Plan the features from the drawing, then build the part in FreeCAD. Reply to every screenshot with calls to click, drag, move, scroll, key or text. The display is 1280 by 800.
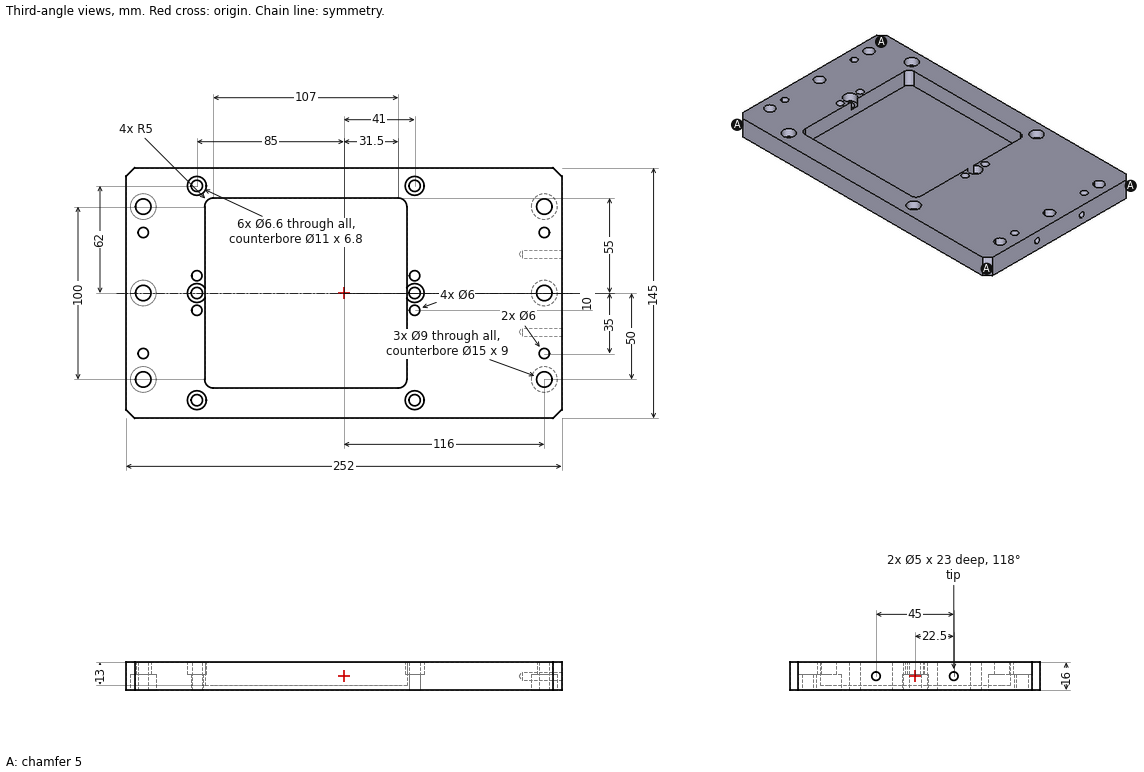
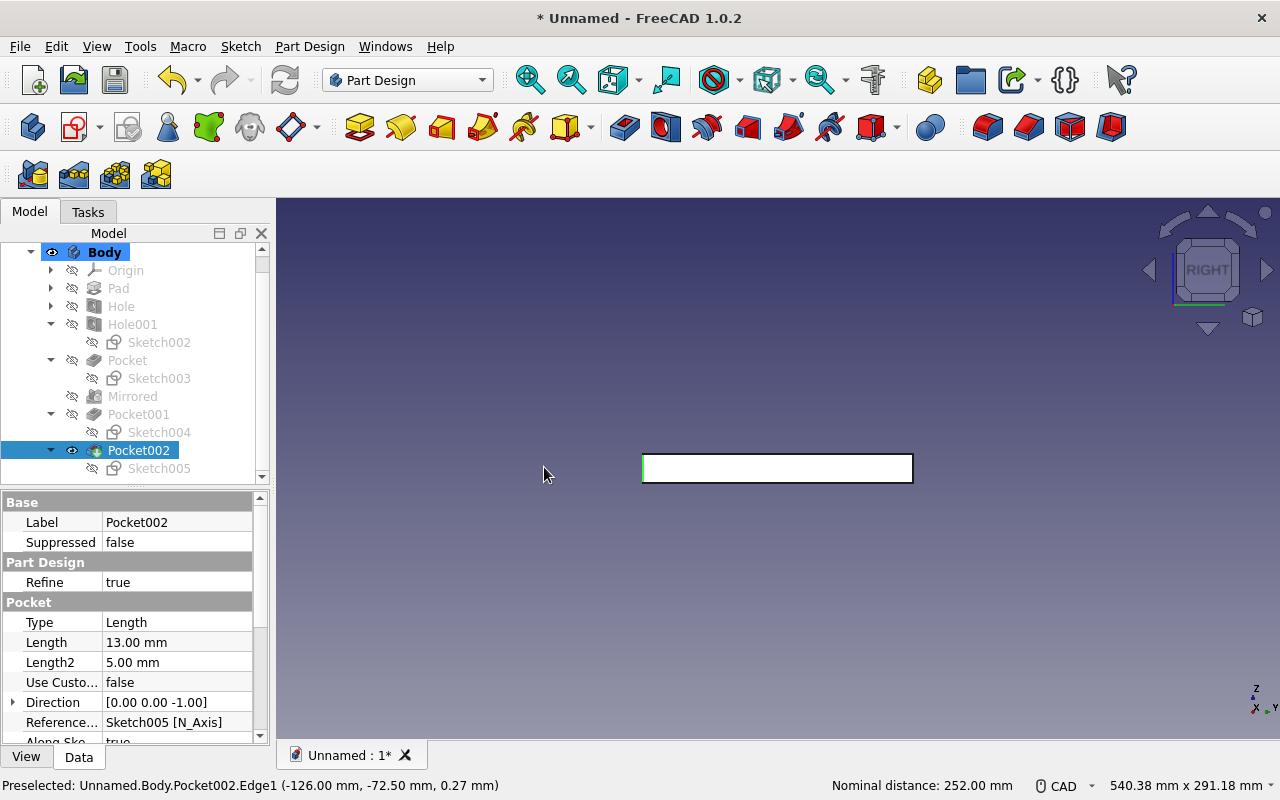
key(v)
key(f)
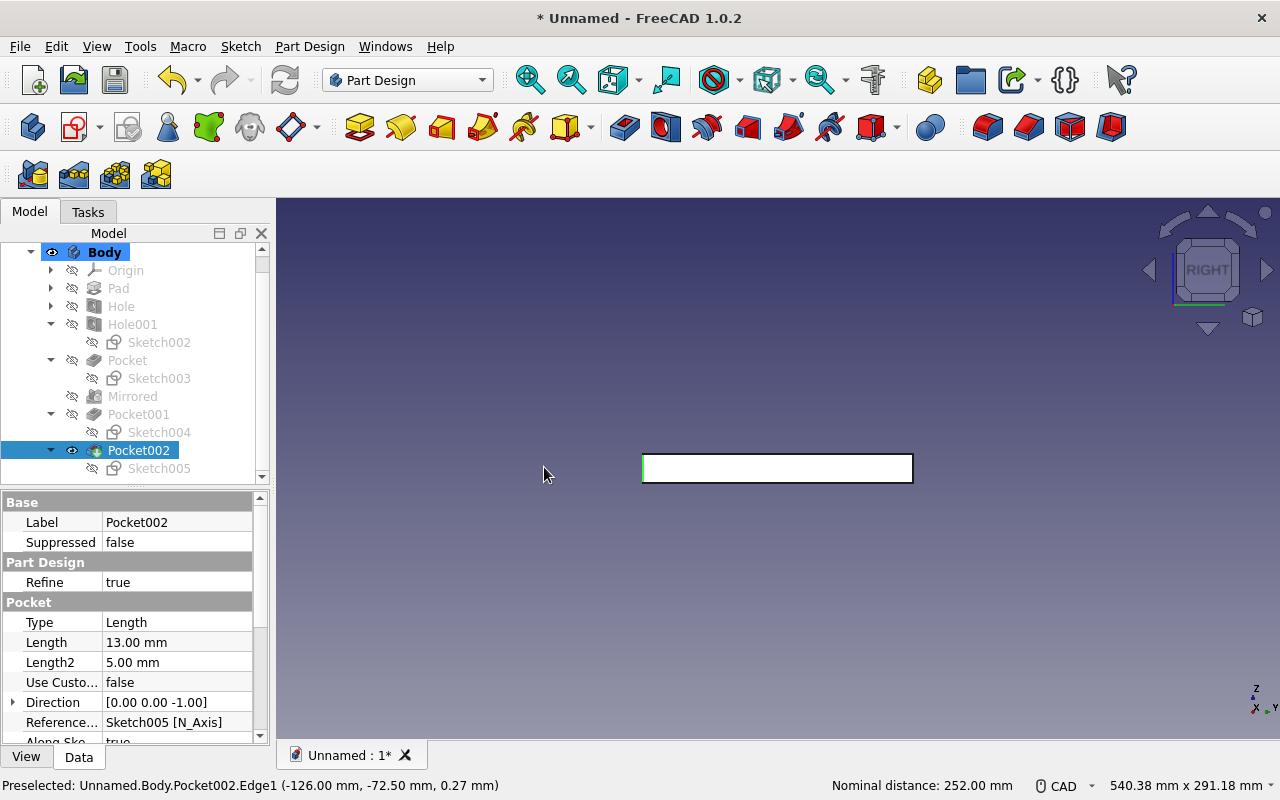
click(913, 467, ctrl)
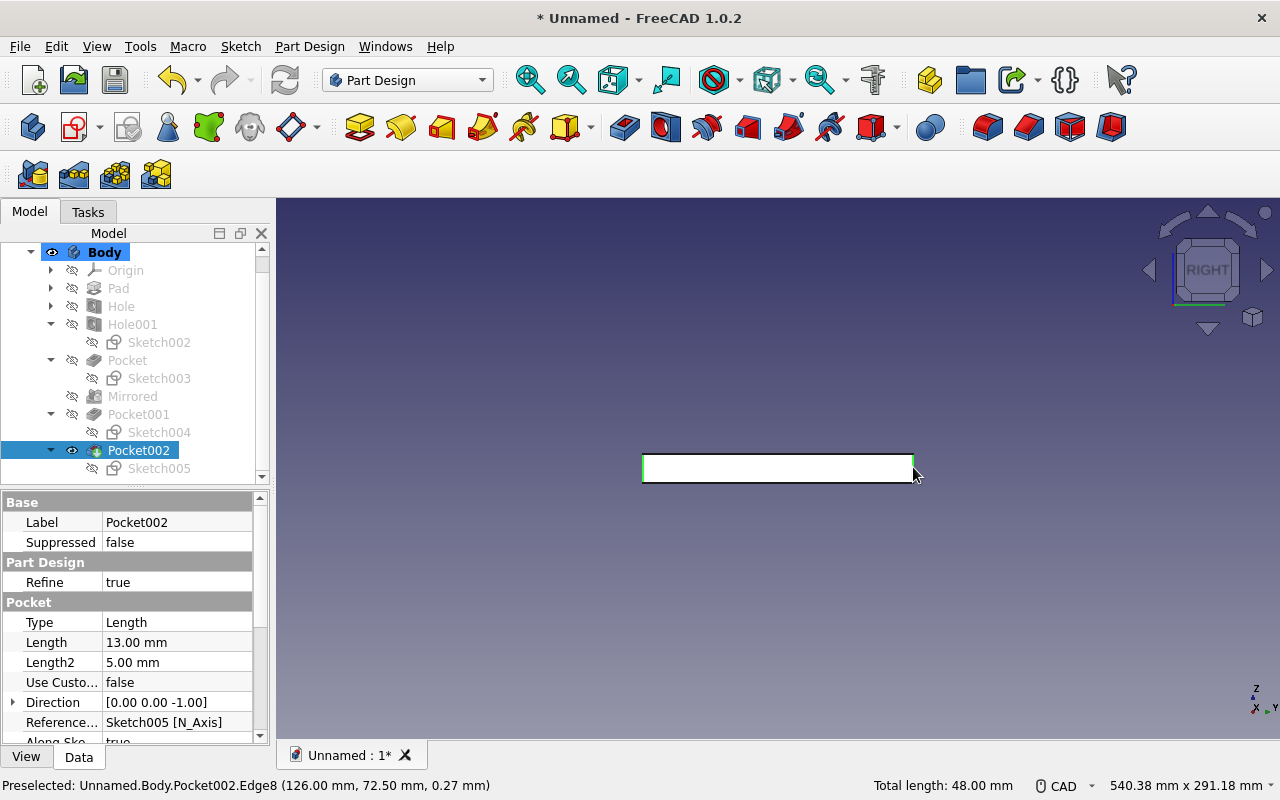
key(5)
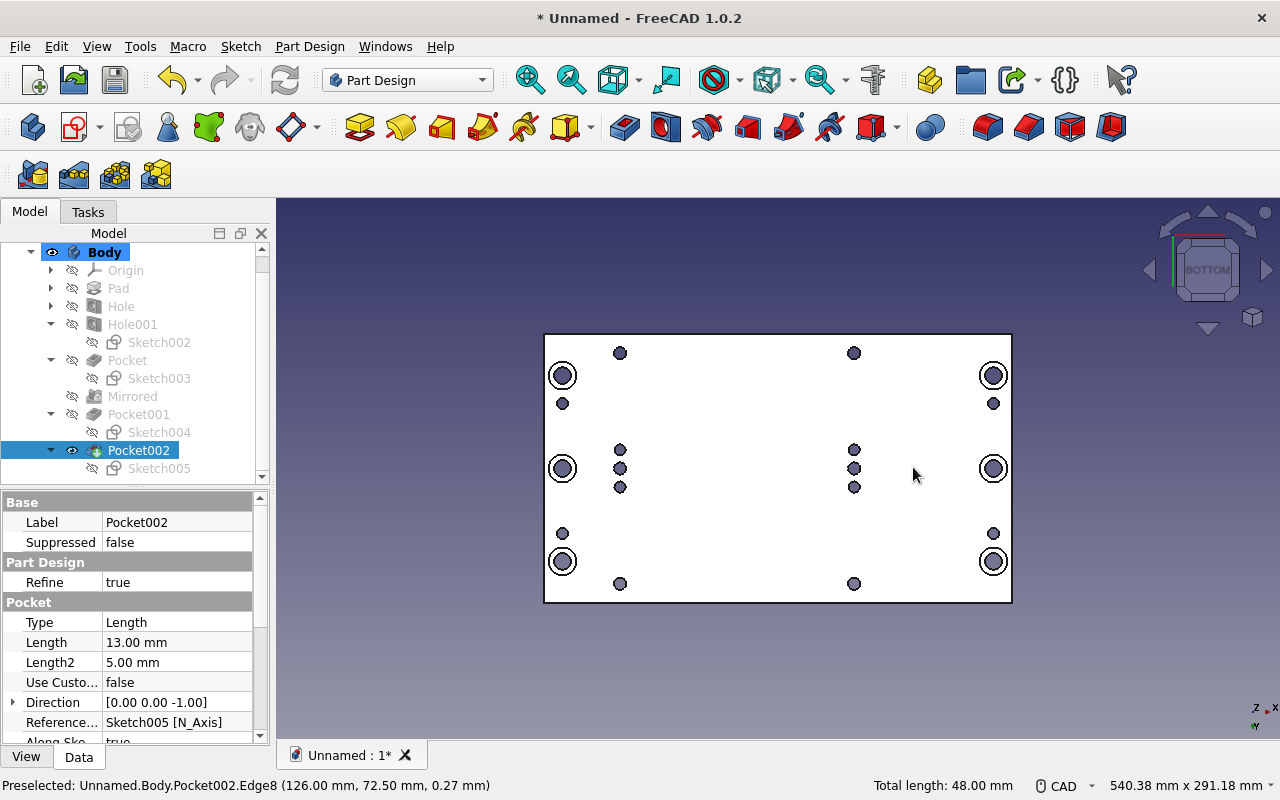
key(4)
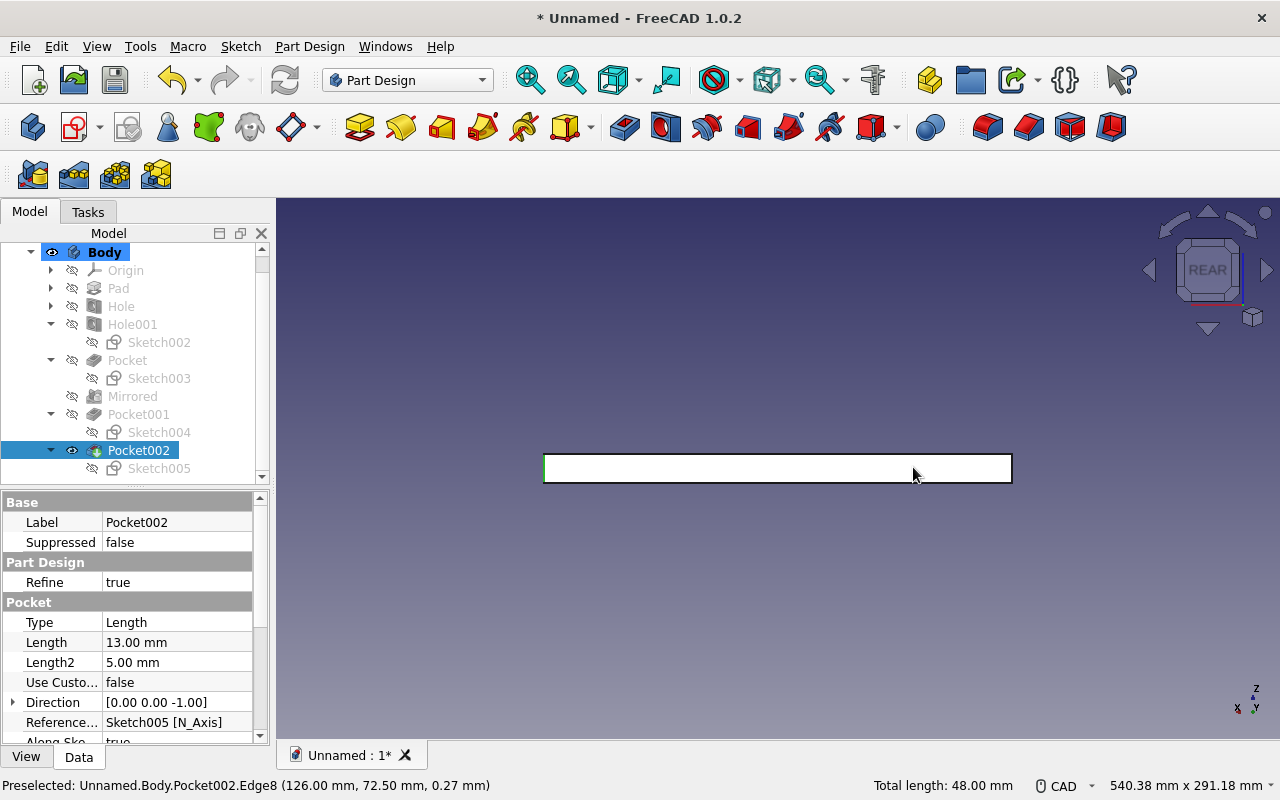
click(1012, 467, ctrl)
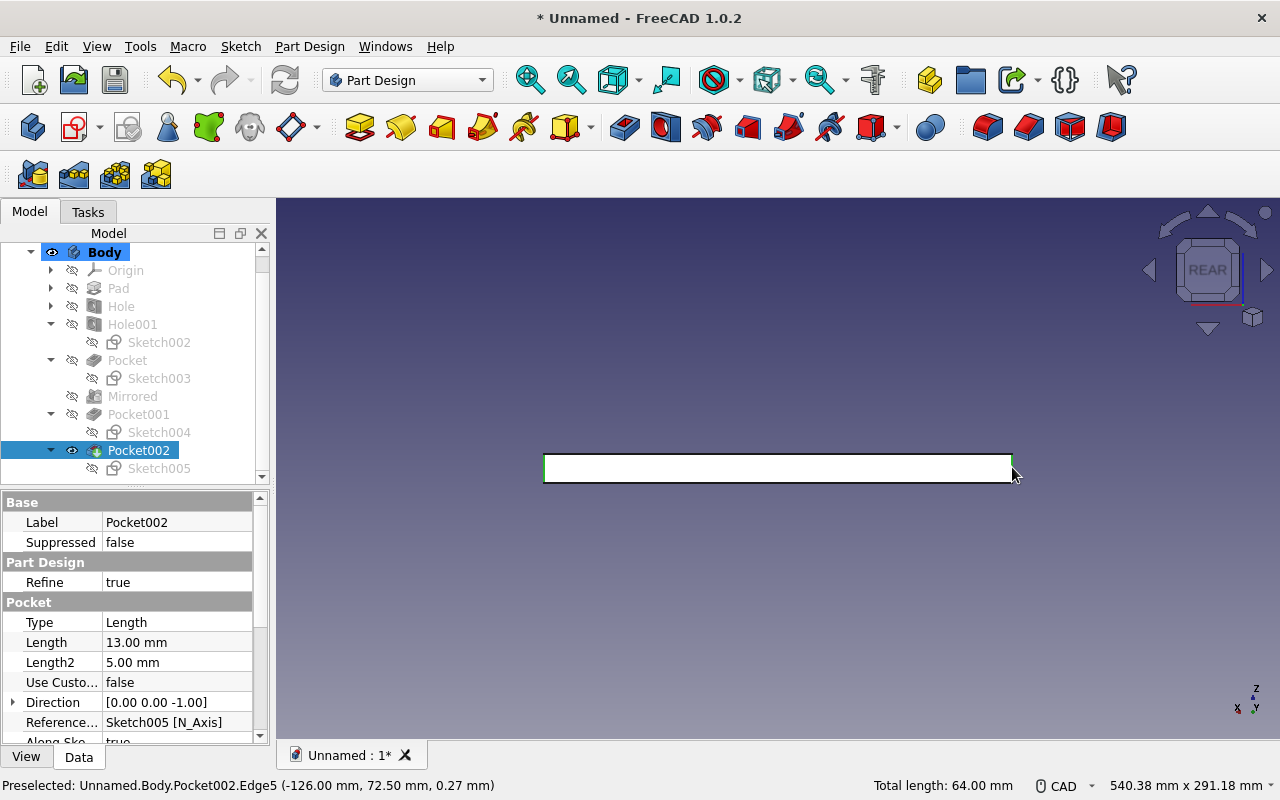
click(1029, 128)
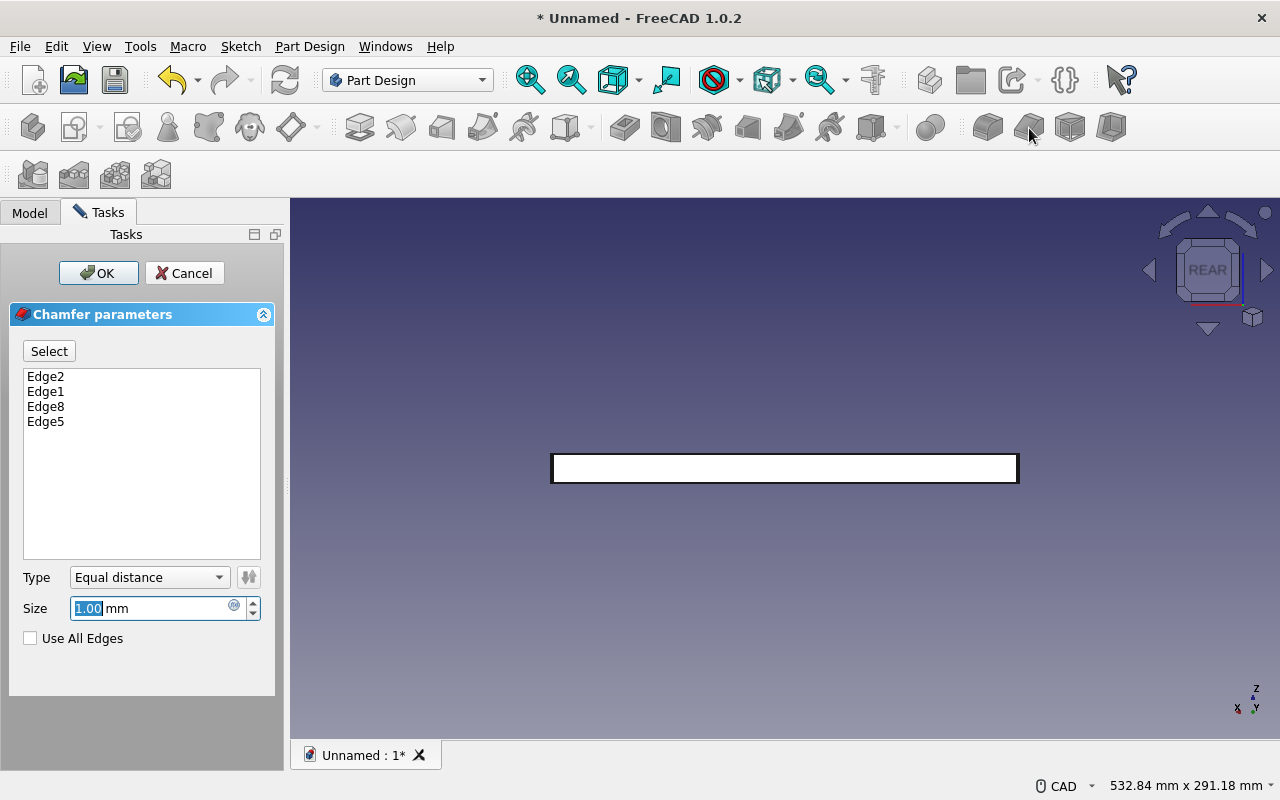
text(5)
key(Tab)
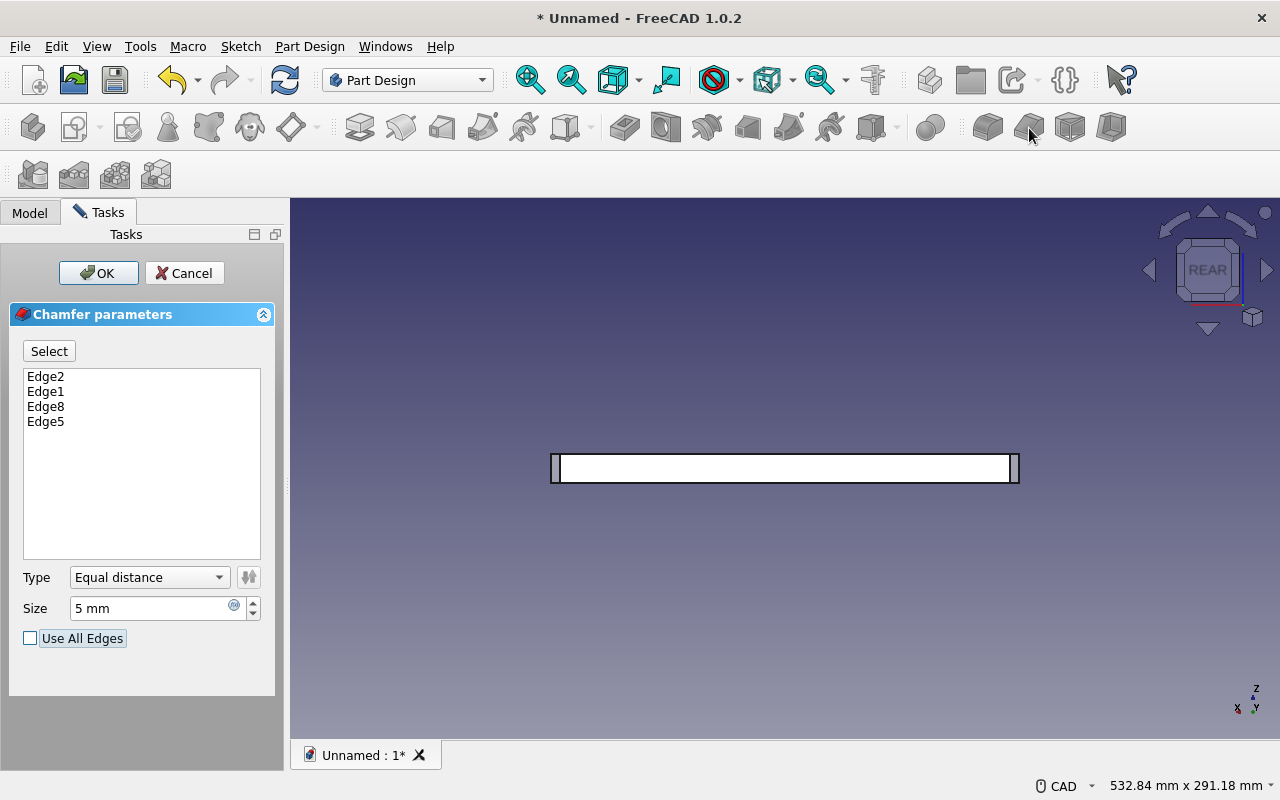
click(99, 273)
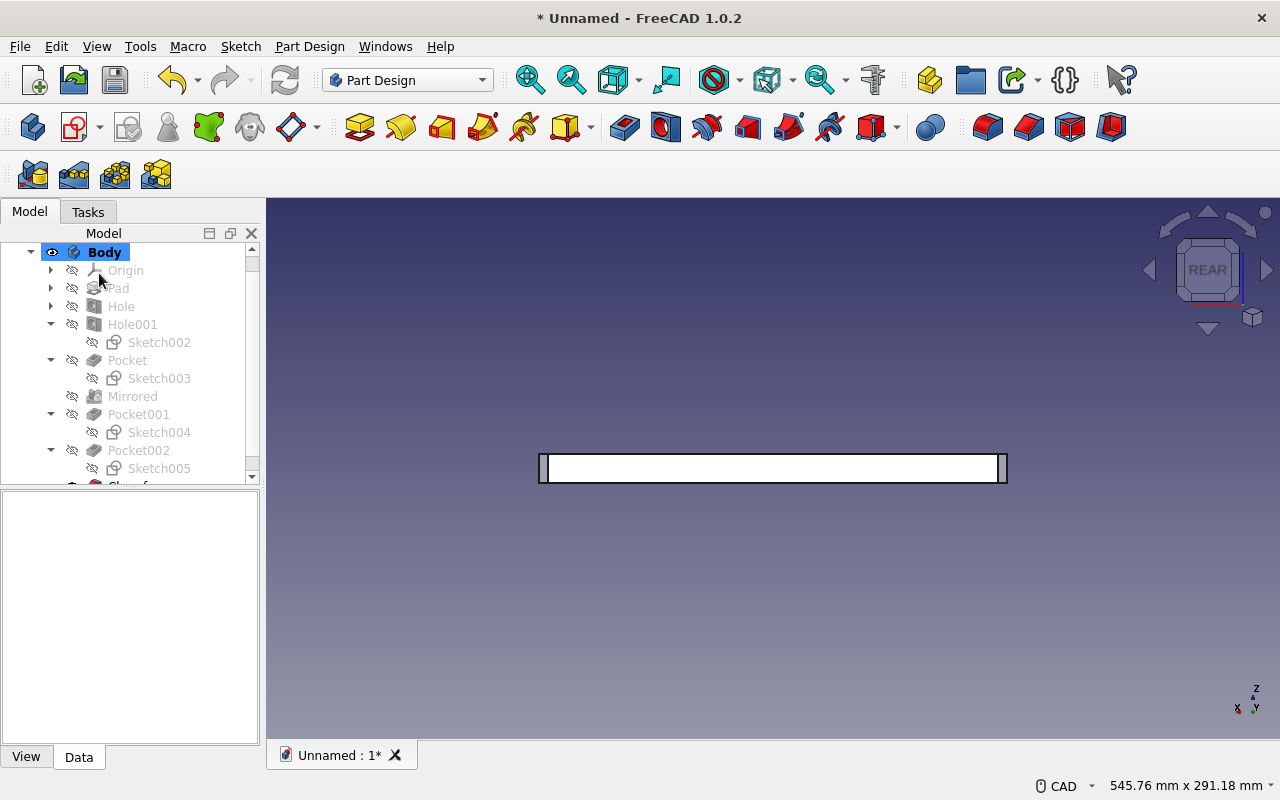
key(0)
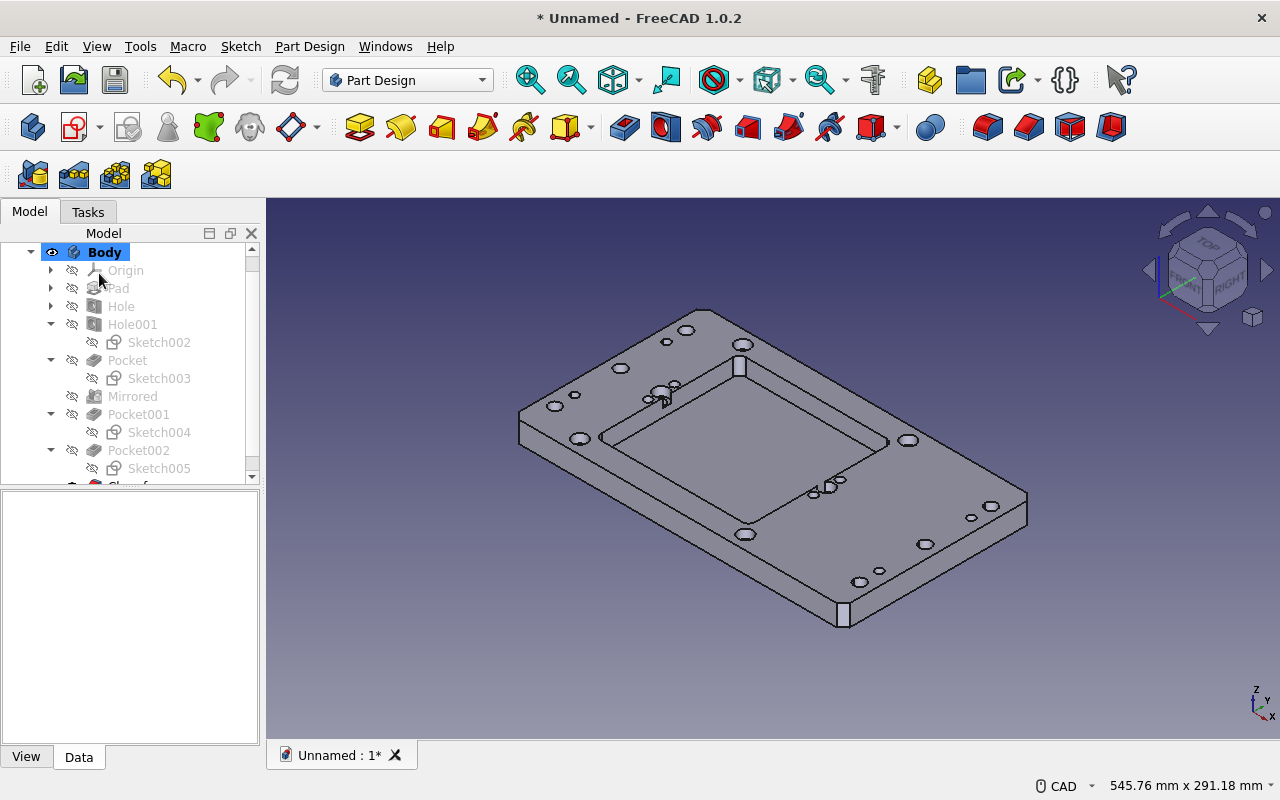
click(1015, 519)